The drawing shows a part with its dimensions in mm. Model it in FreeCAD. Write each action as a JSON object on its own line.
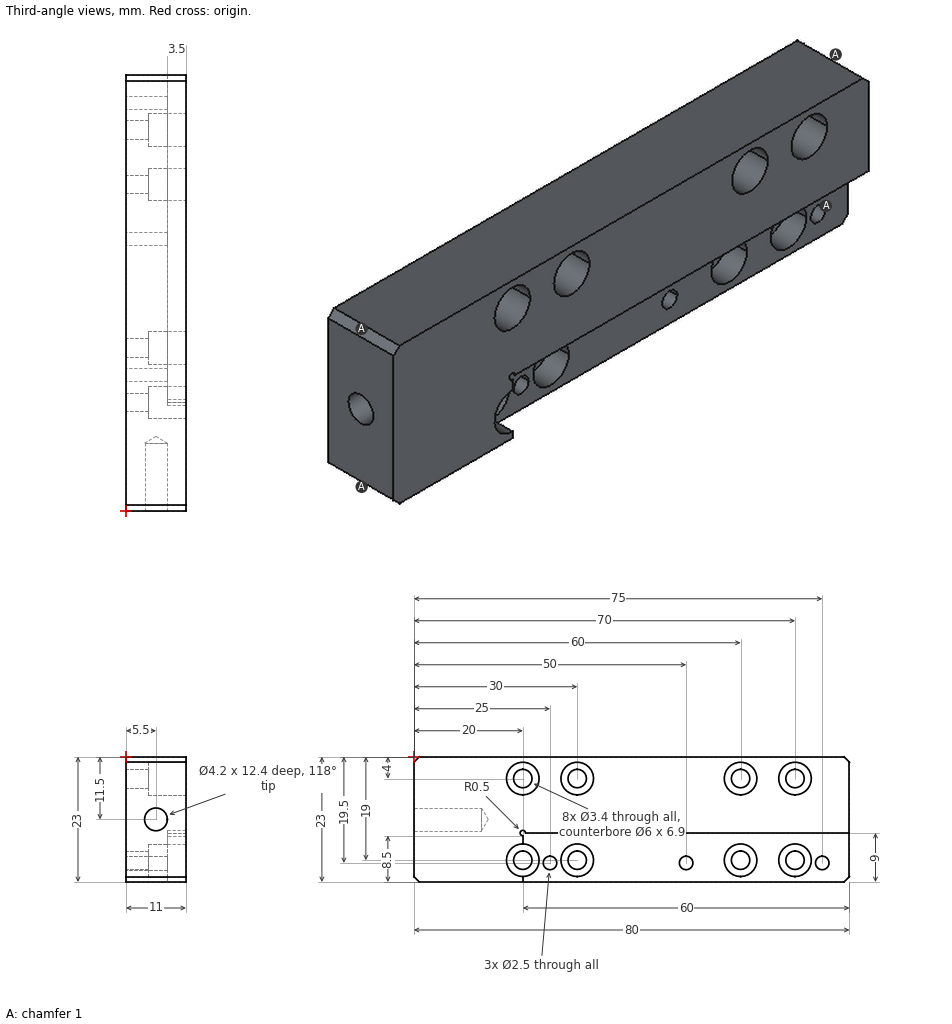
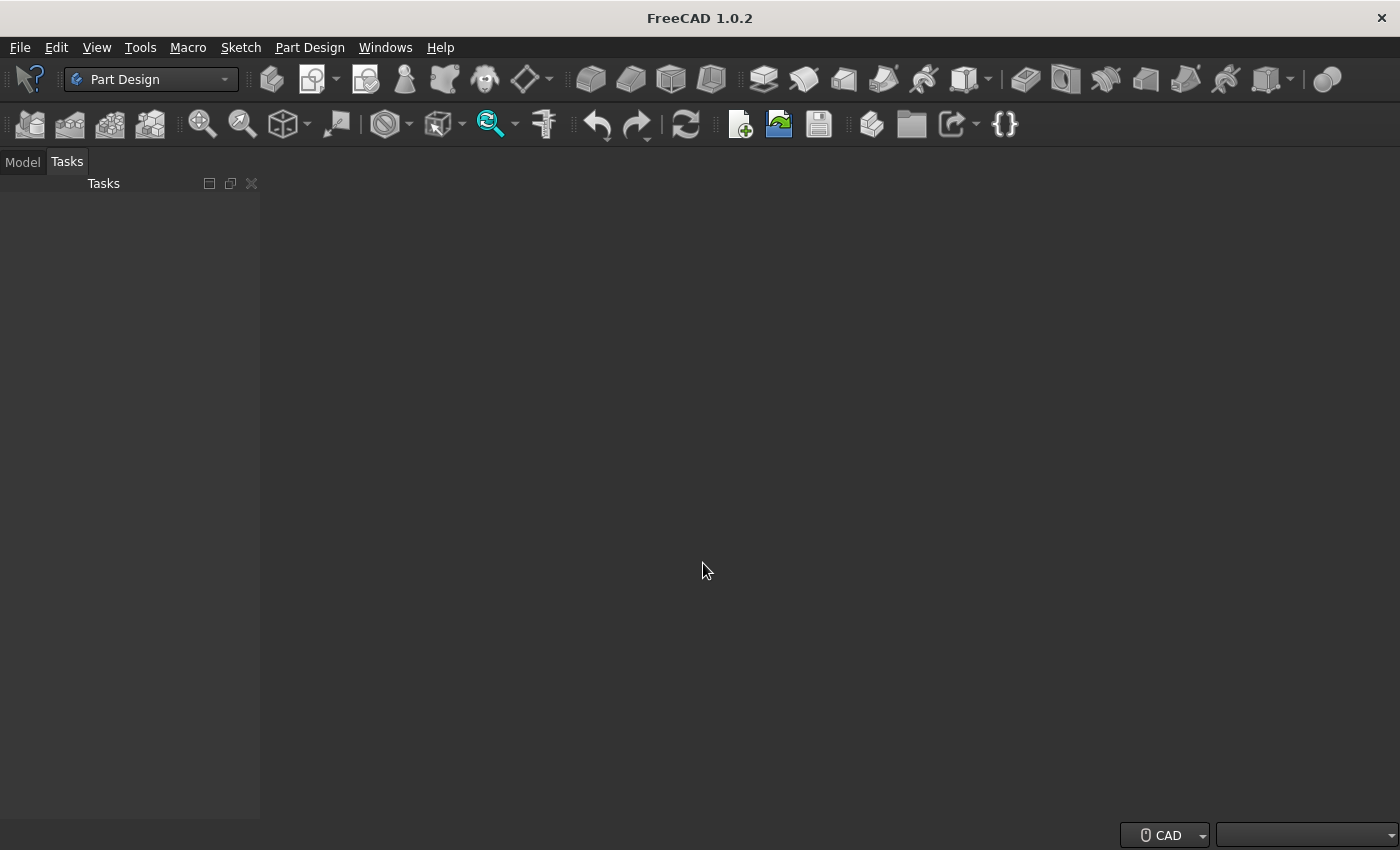
{"action": "left_click", "coordinate": [740, 124]}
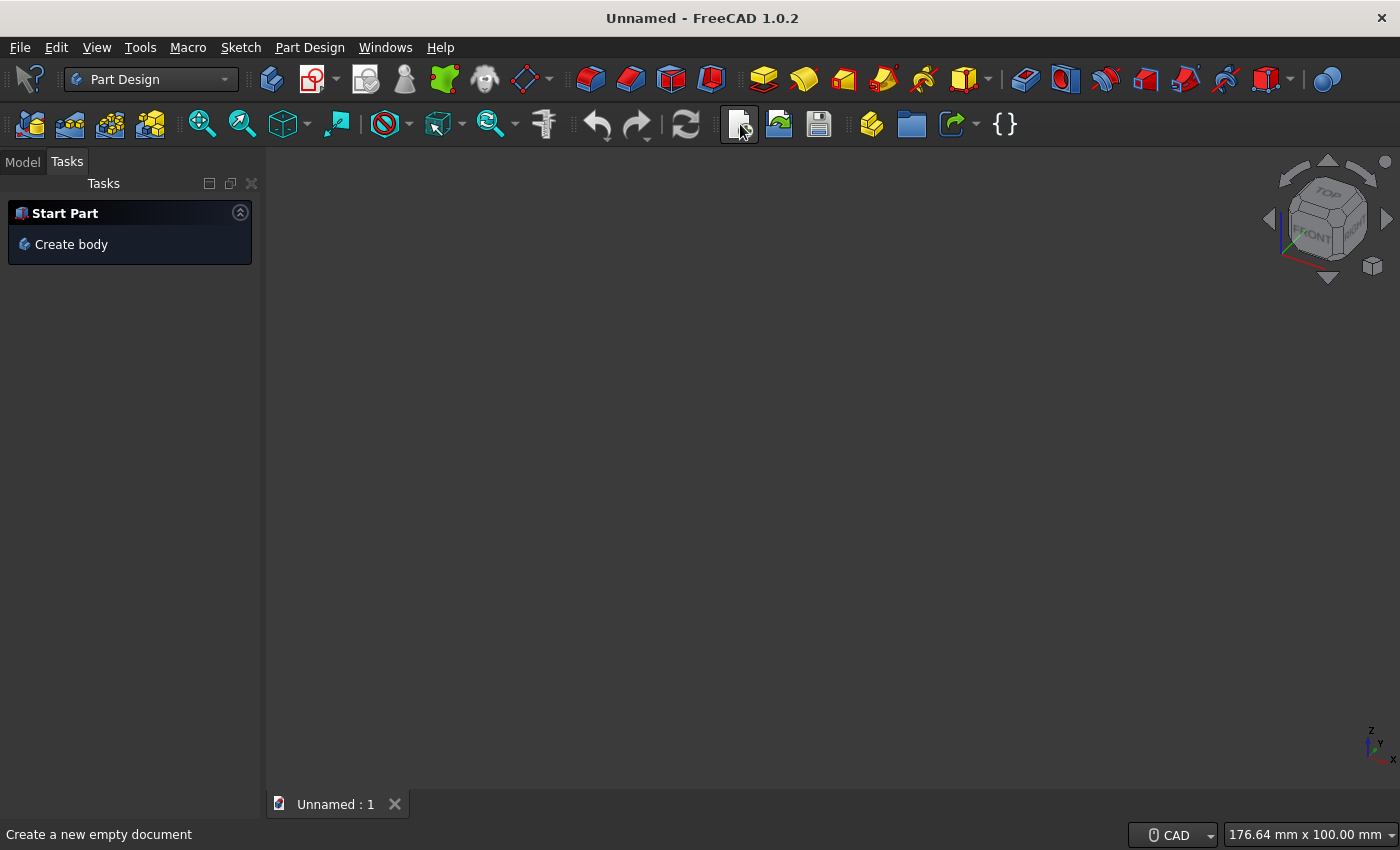
{"action": "left_click", "coordinate": [312, 80]}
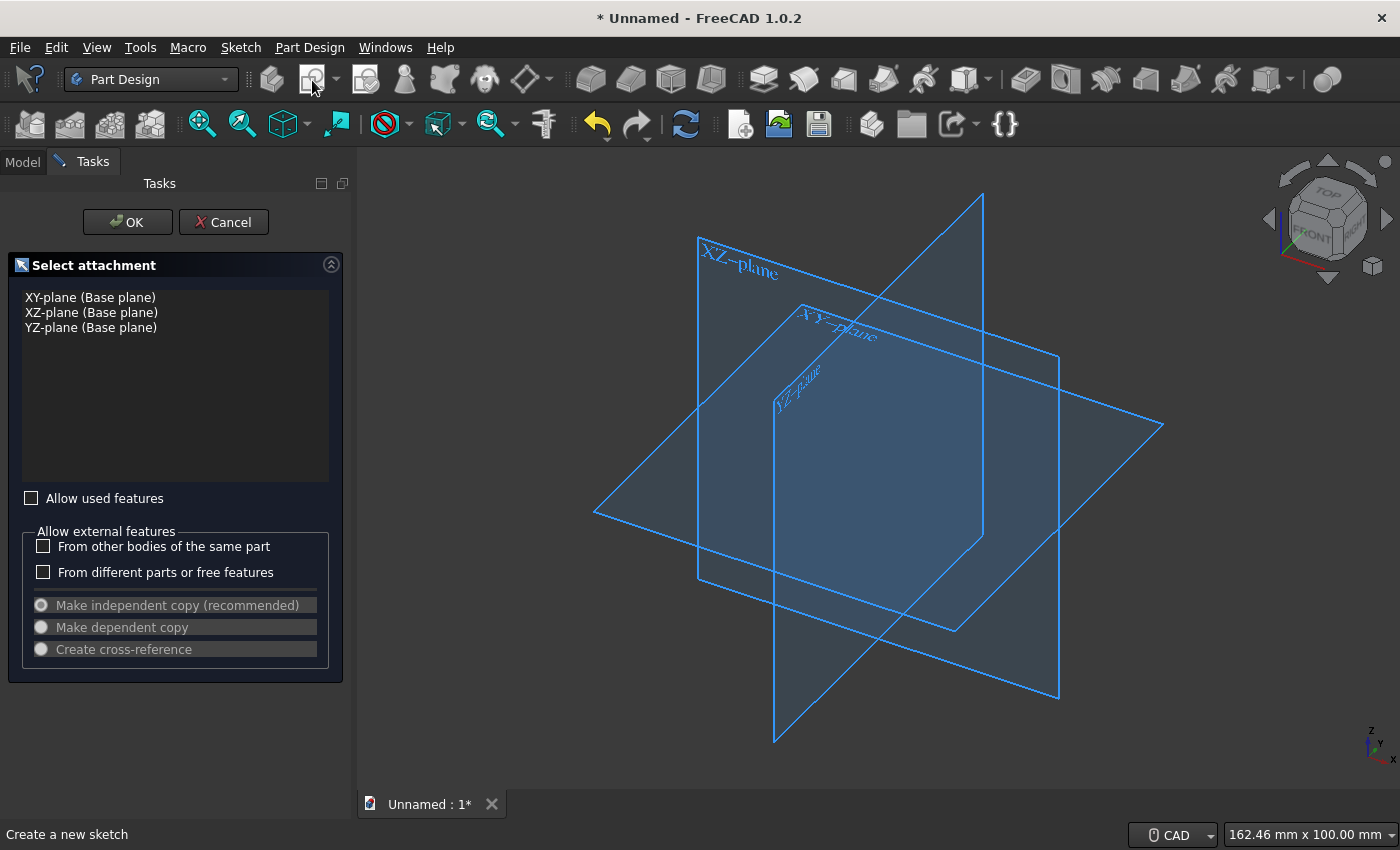
{"action": "left_click", "coordinate": [82, 312]}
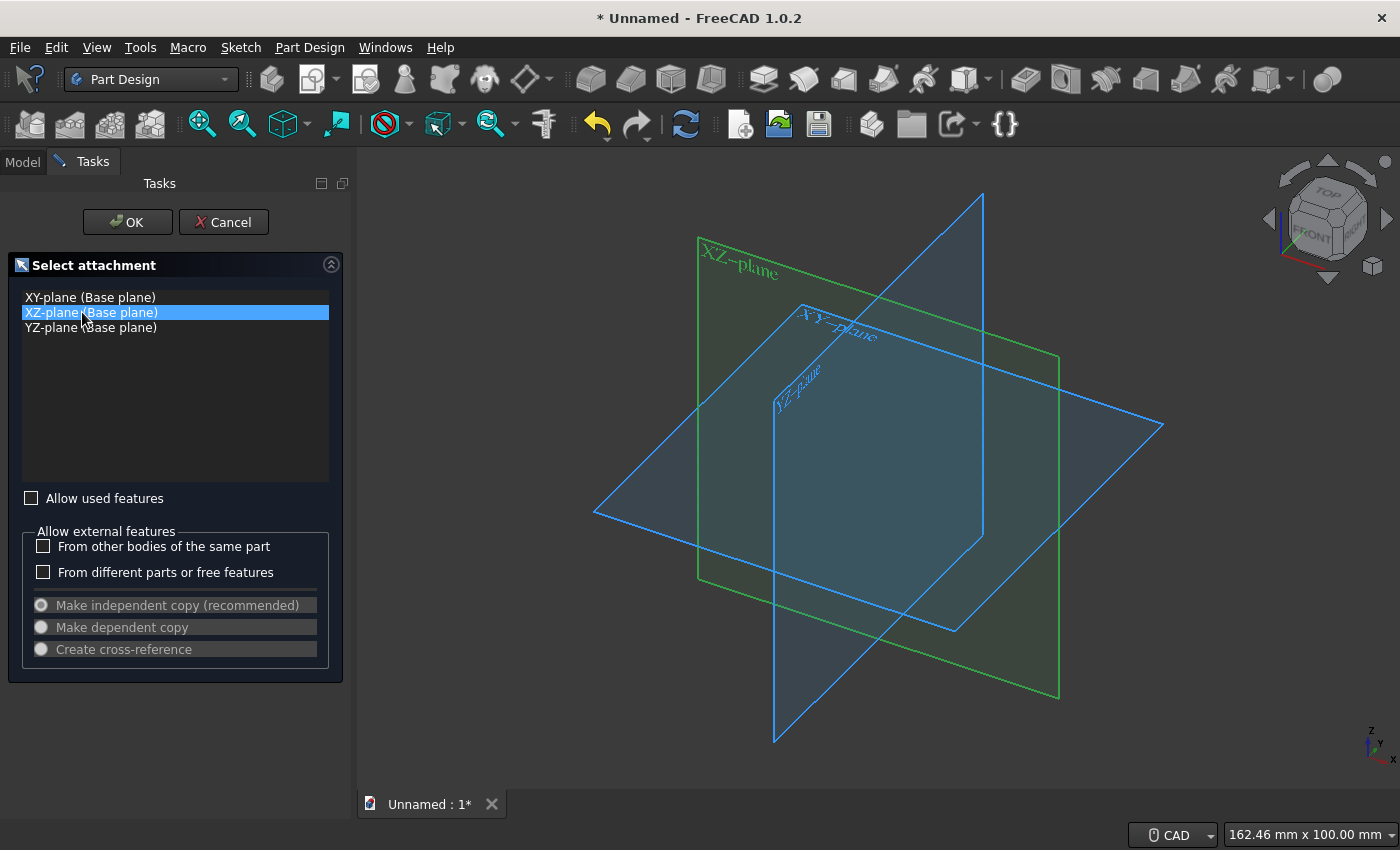
{"action": "left_click", "coordinate": [128, 222]}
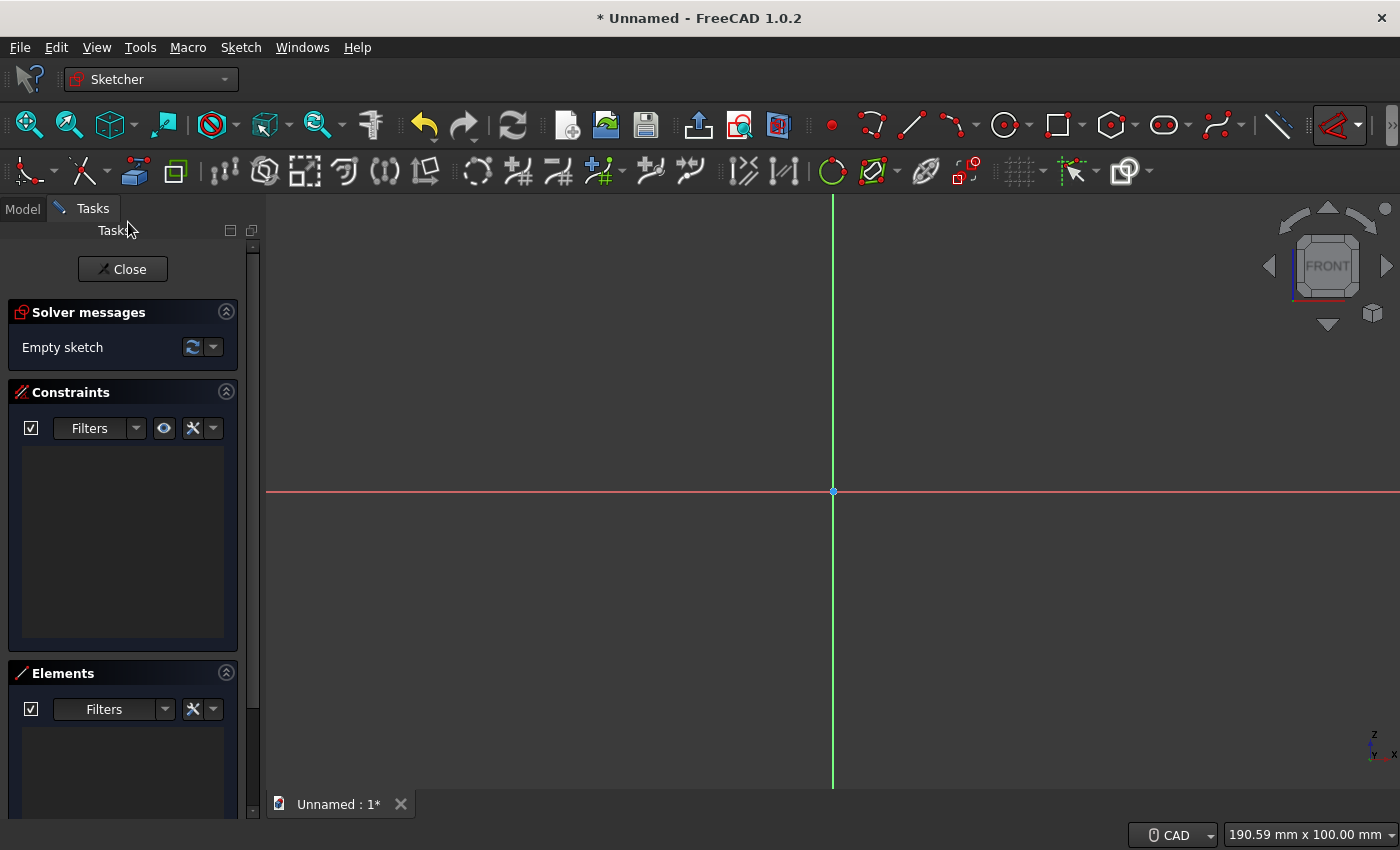
{"action": "scroll", "coordinate": [925, 600], "scroll_direction": "up", "scroll_amount": 5}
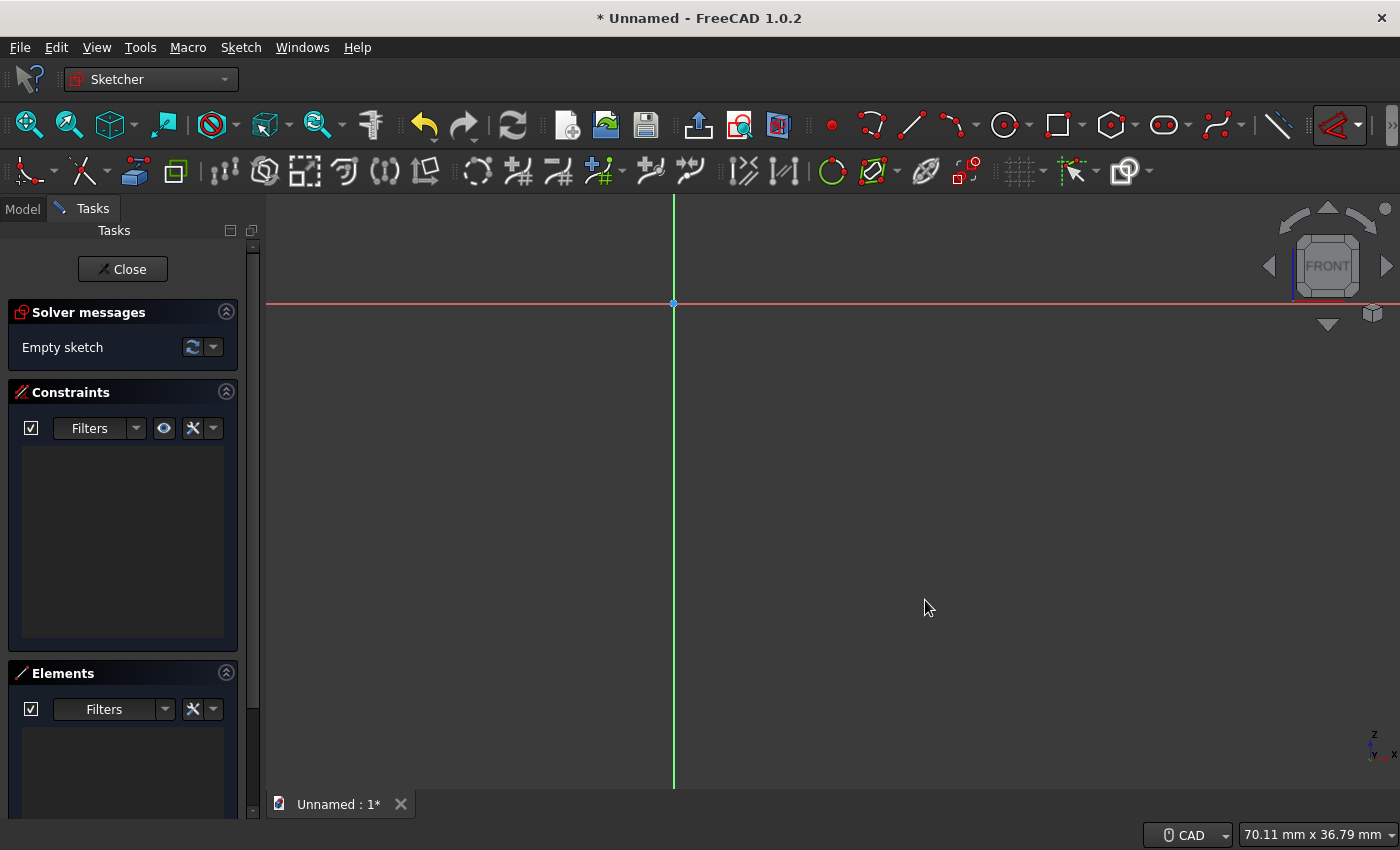
{"action": "left_click", "coordinate": [1058, 126]}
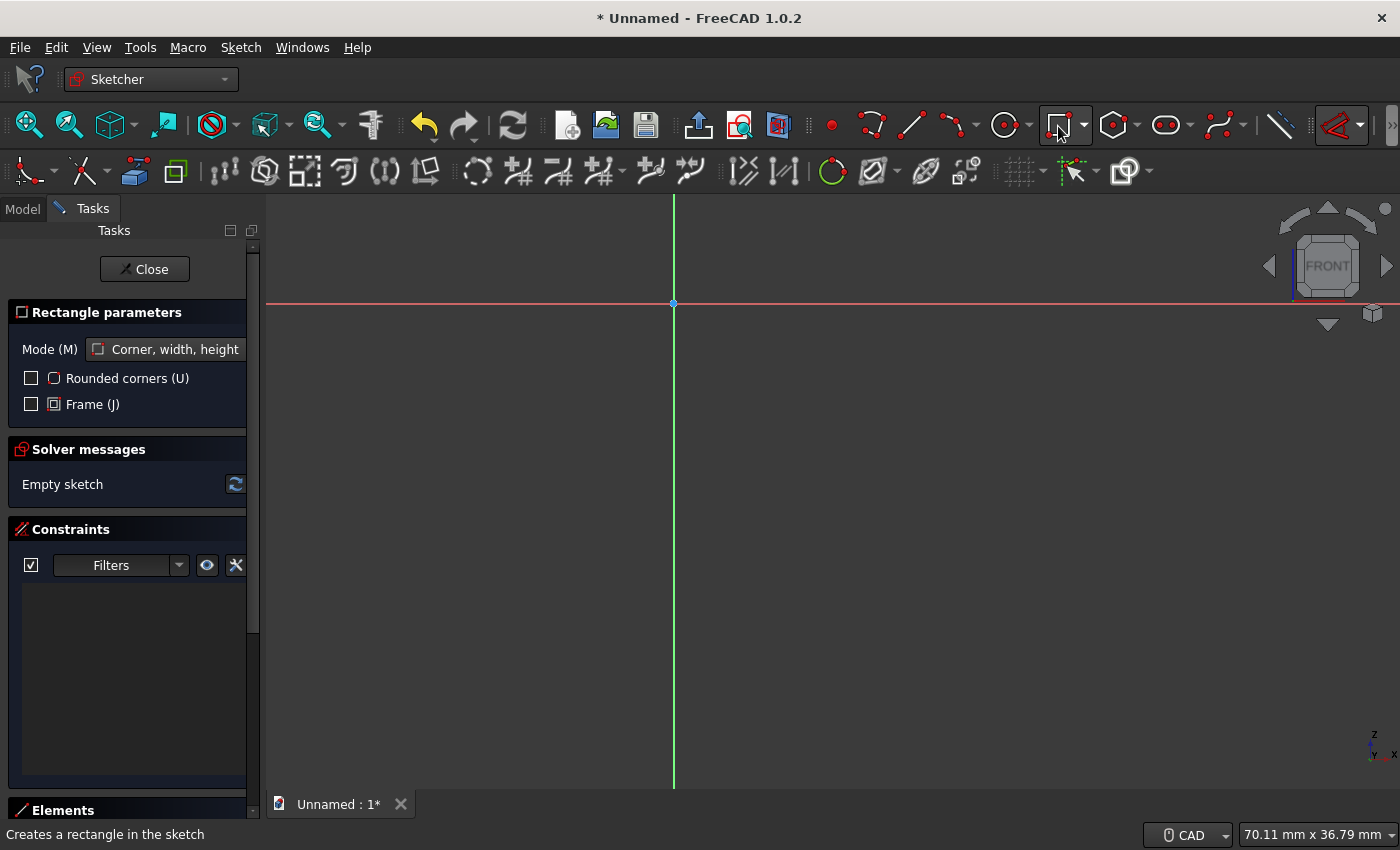
{"action": "left_click", "coordinate": [674, 304]}
{"action": "left_click", "coordinate": [852, 676]}
{"action": "key", "text": "Escape"}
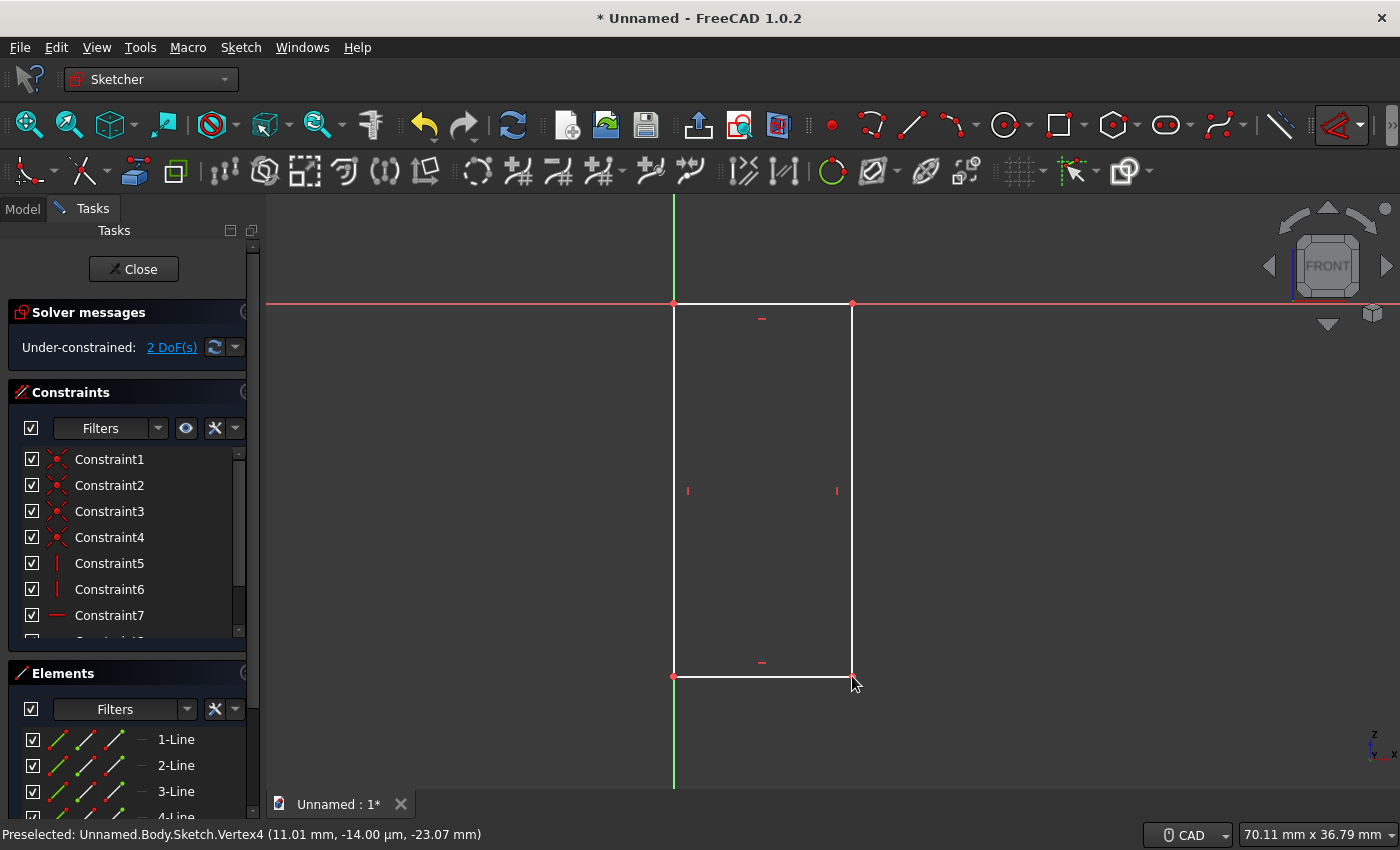
{"action": "left_click", "coordinate": [1336, 126]}